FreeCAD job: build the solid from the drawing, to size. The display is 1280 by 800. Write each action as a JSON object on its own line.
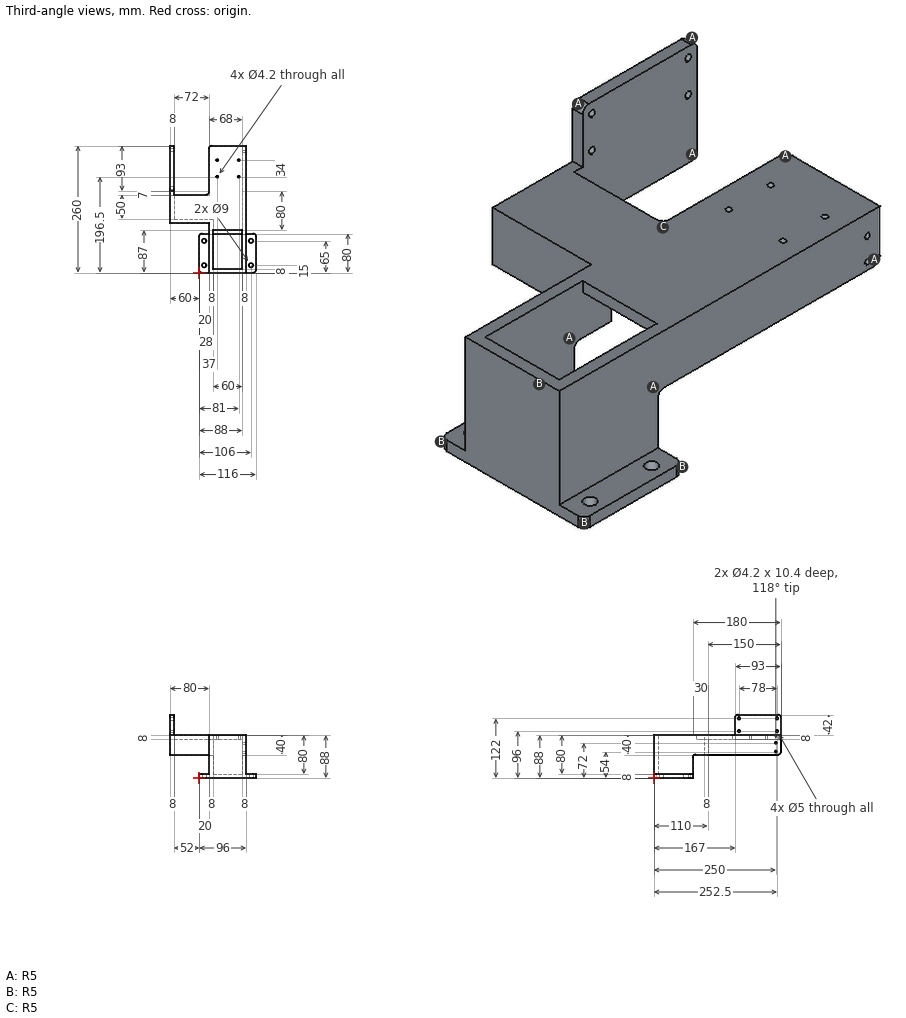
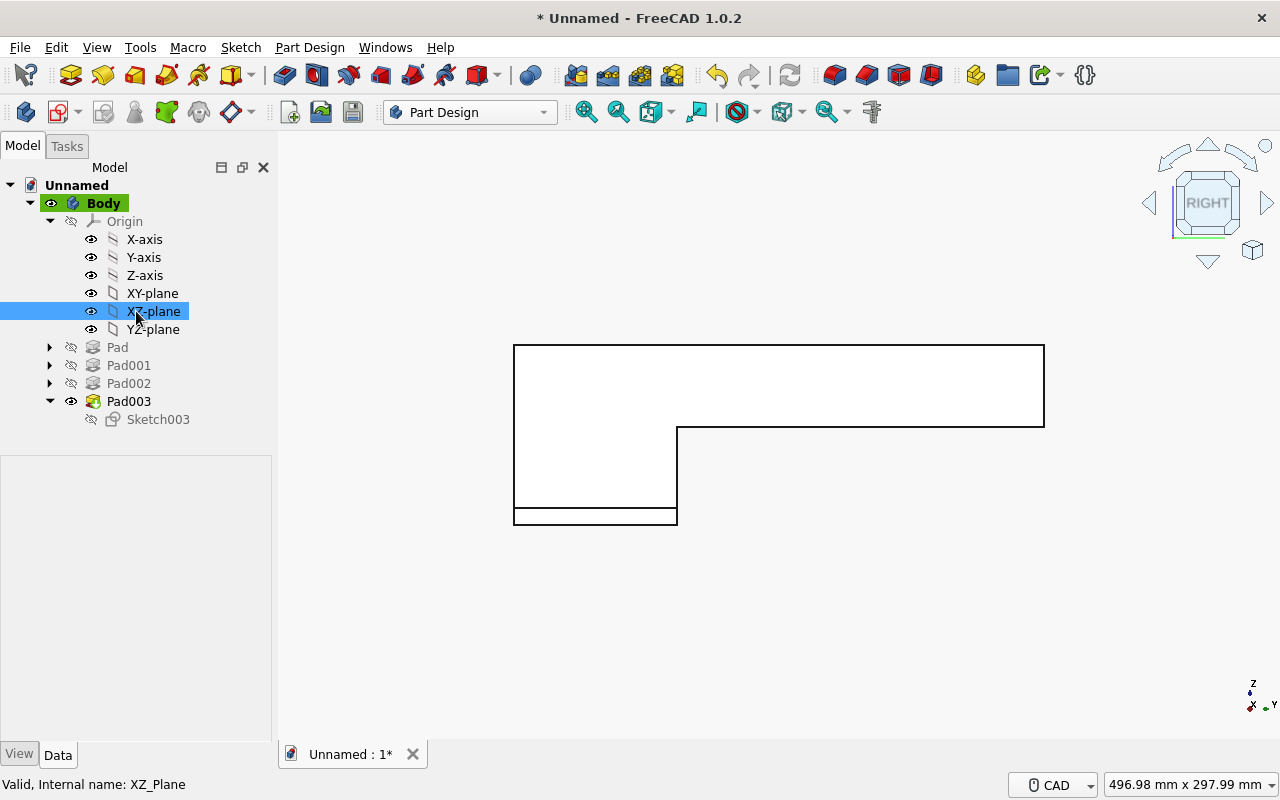
{"action": "left_click", "coordinate": [232, 112]}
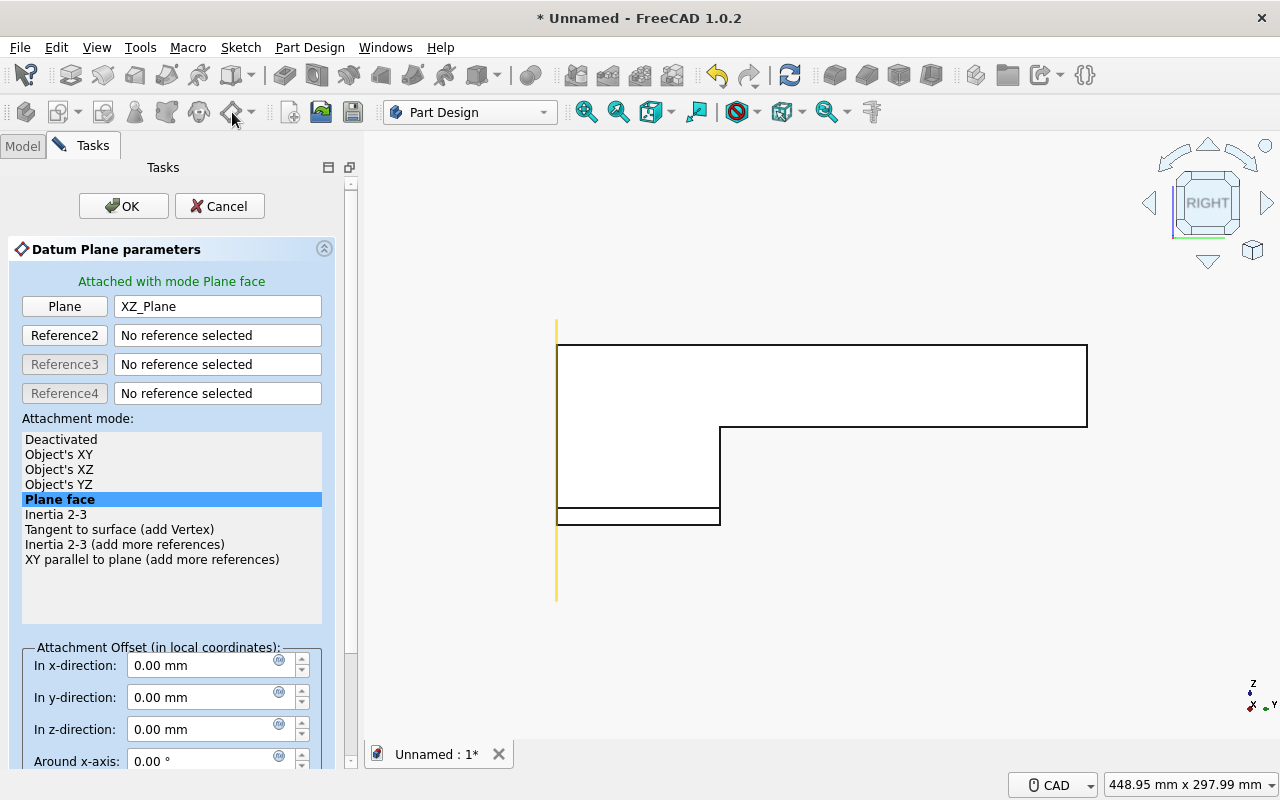
{"action": "triple_click", "coordinate": [210, 729]}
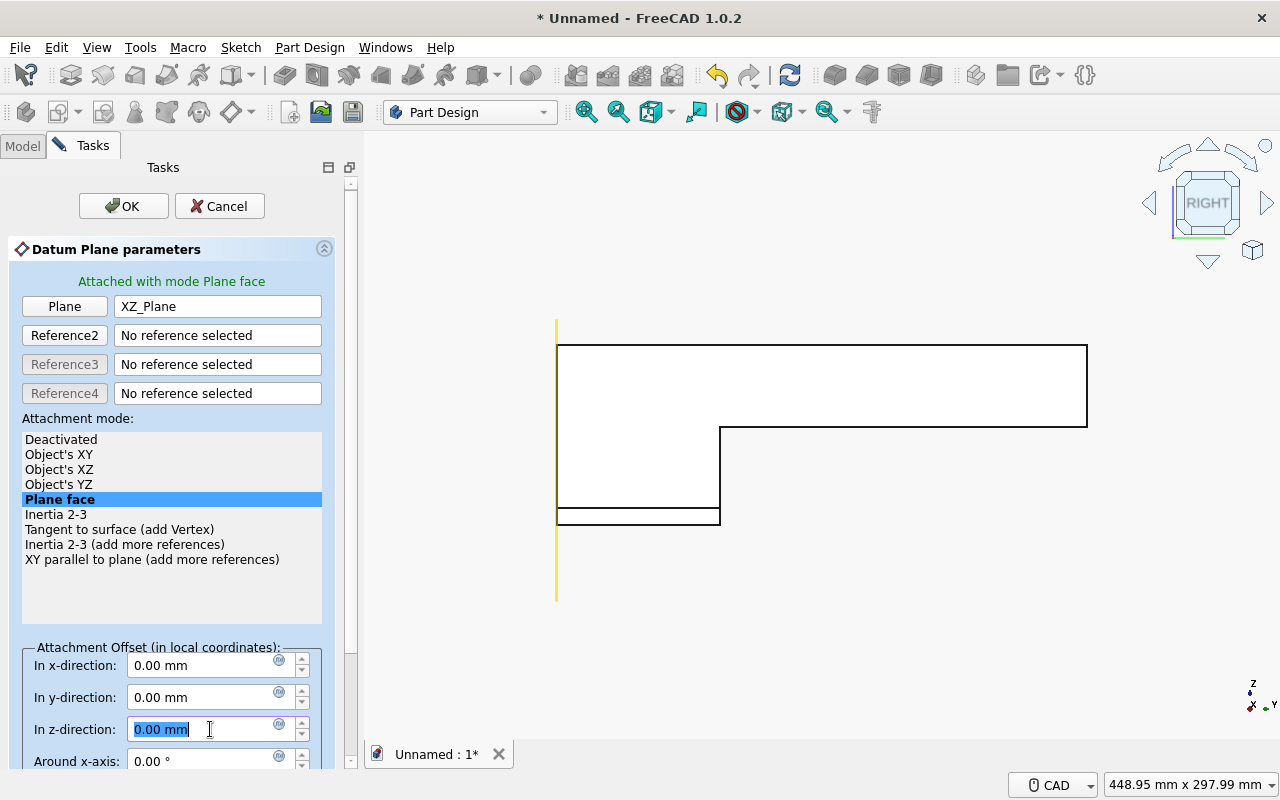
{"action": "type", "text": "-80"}
{"action": "key", "text": "Tab"}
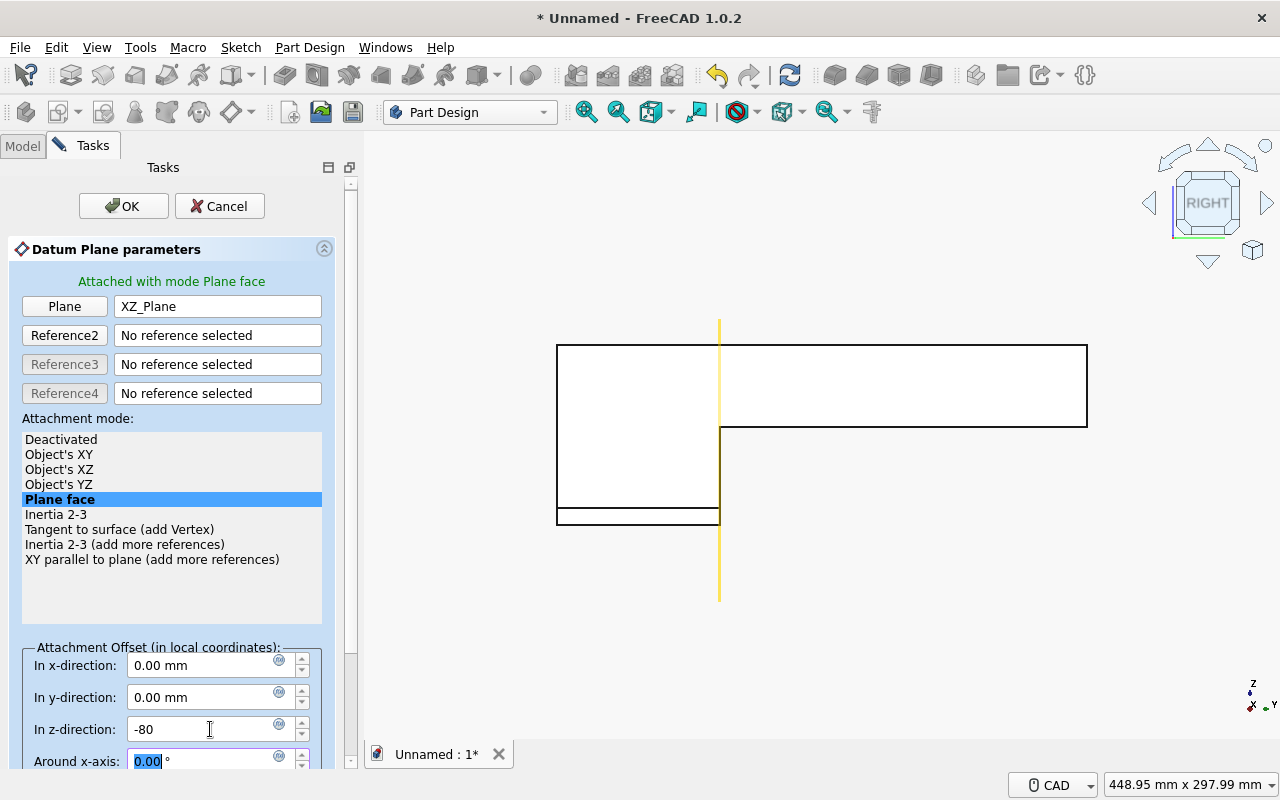
{"action": "left_click", "coordinate": [124, 206]}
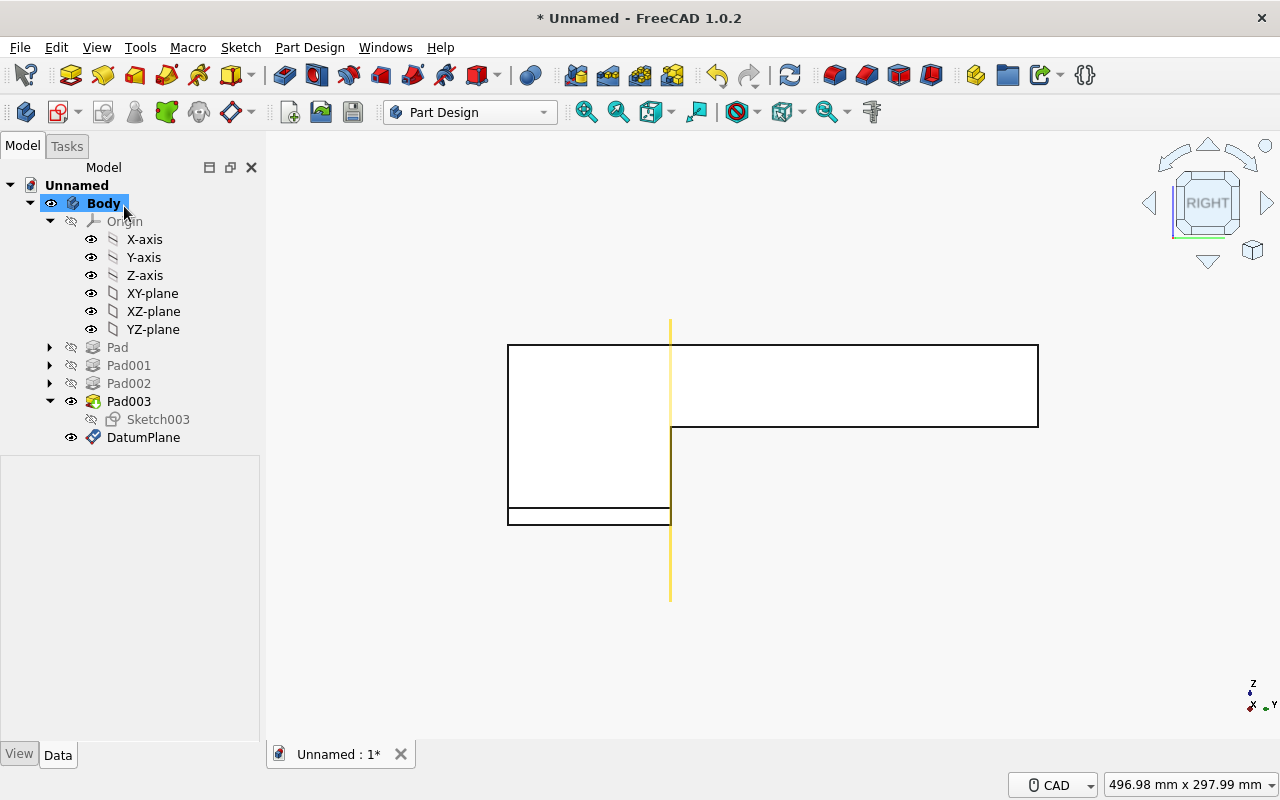
{"action": "left_click", "coordinate": [116, 437]}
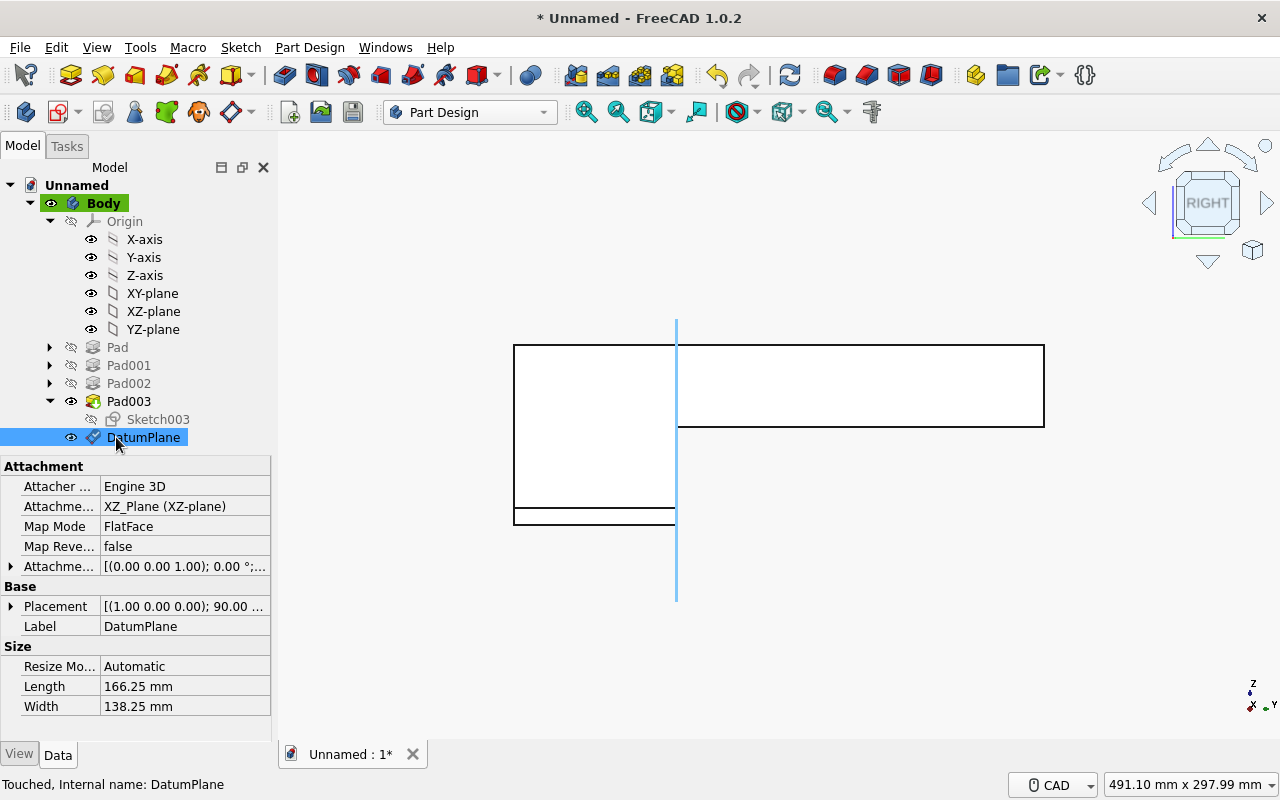
{"action": "left_click", "coordinate": [58, 112]}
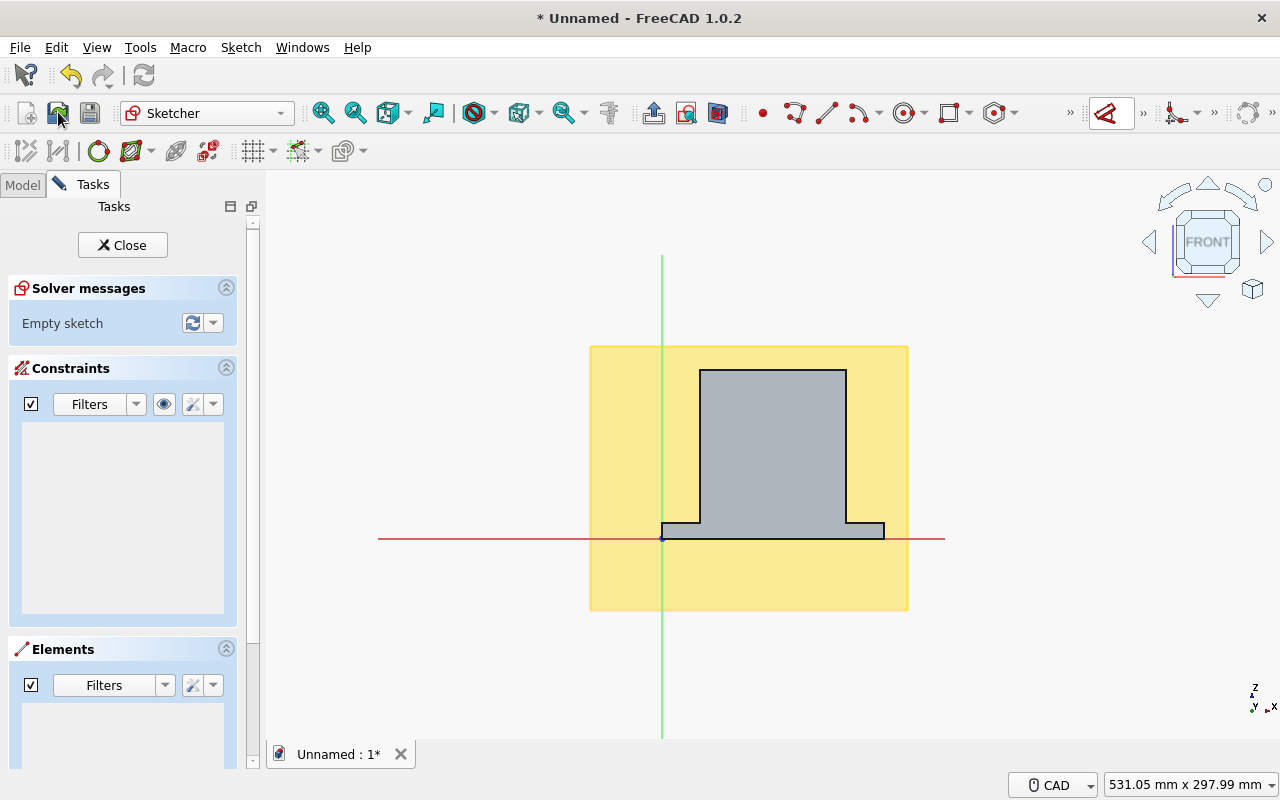
{"action": "left_click", "coordinate": [718, 114]}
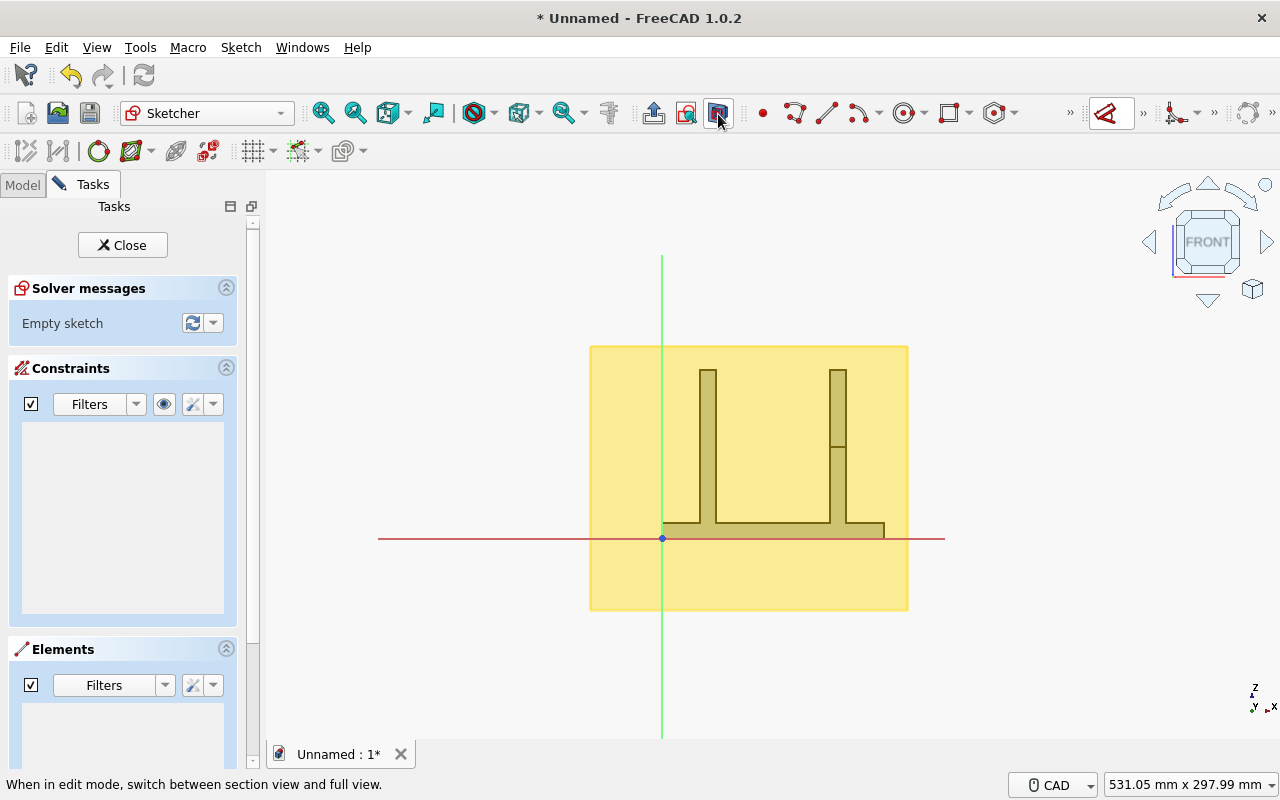
{"action": "scroll", "coordinate": [676, 455], "scroll_direction": "up", "scroll_amount": 4}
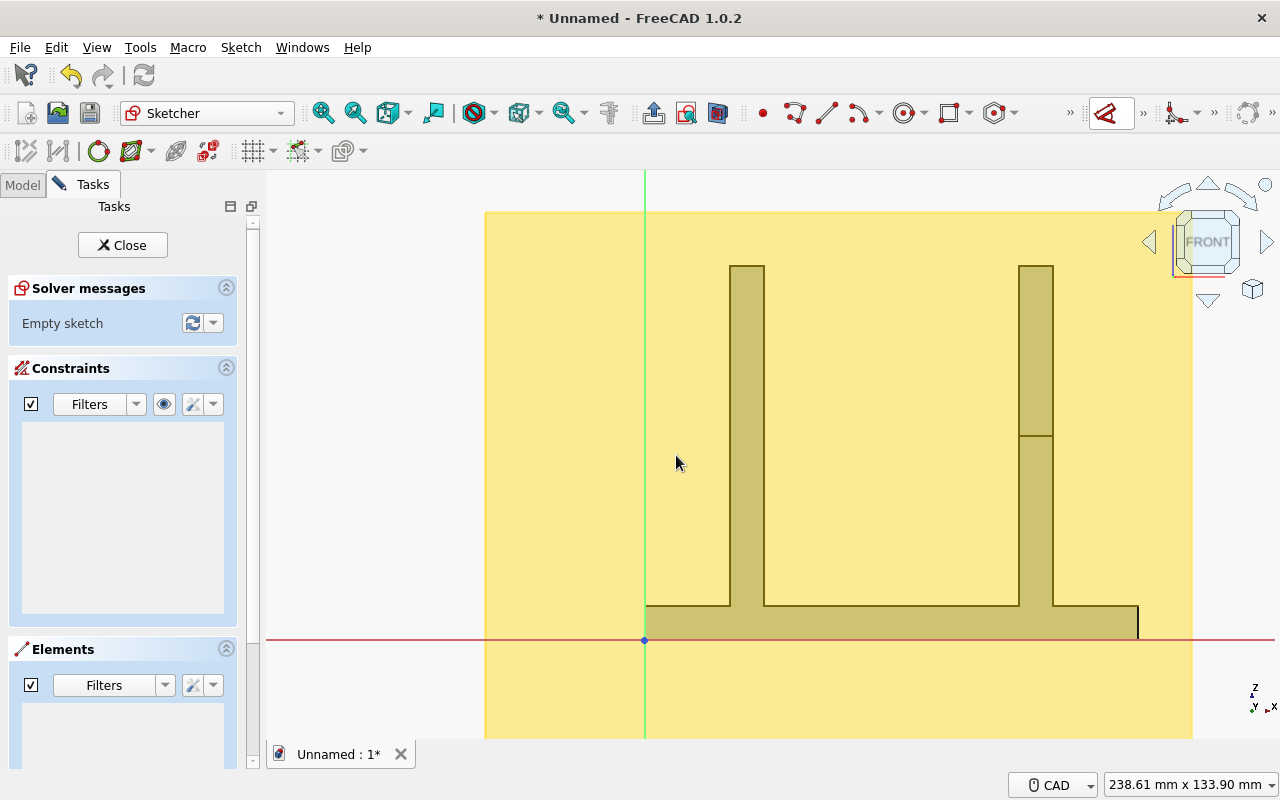
{"action": "left_click", "coordinate": [950, 114]}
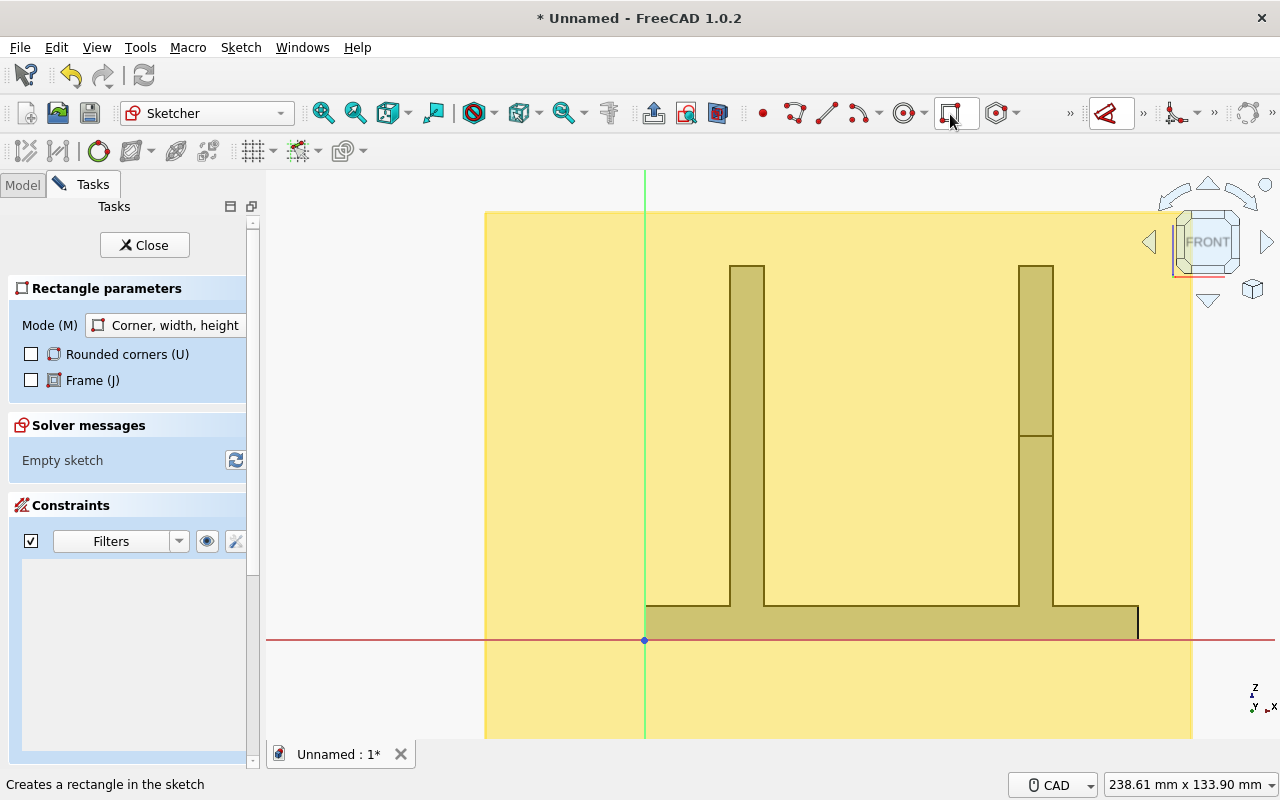
{"action": "left_click", "coordinate": [730, 266]}
{"action": "left_click", "coordinate": [764, 436]}
{"action": "key", "text": "Escape"}